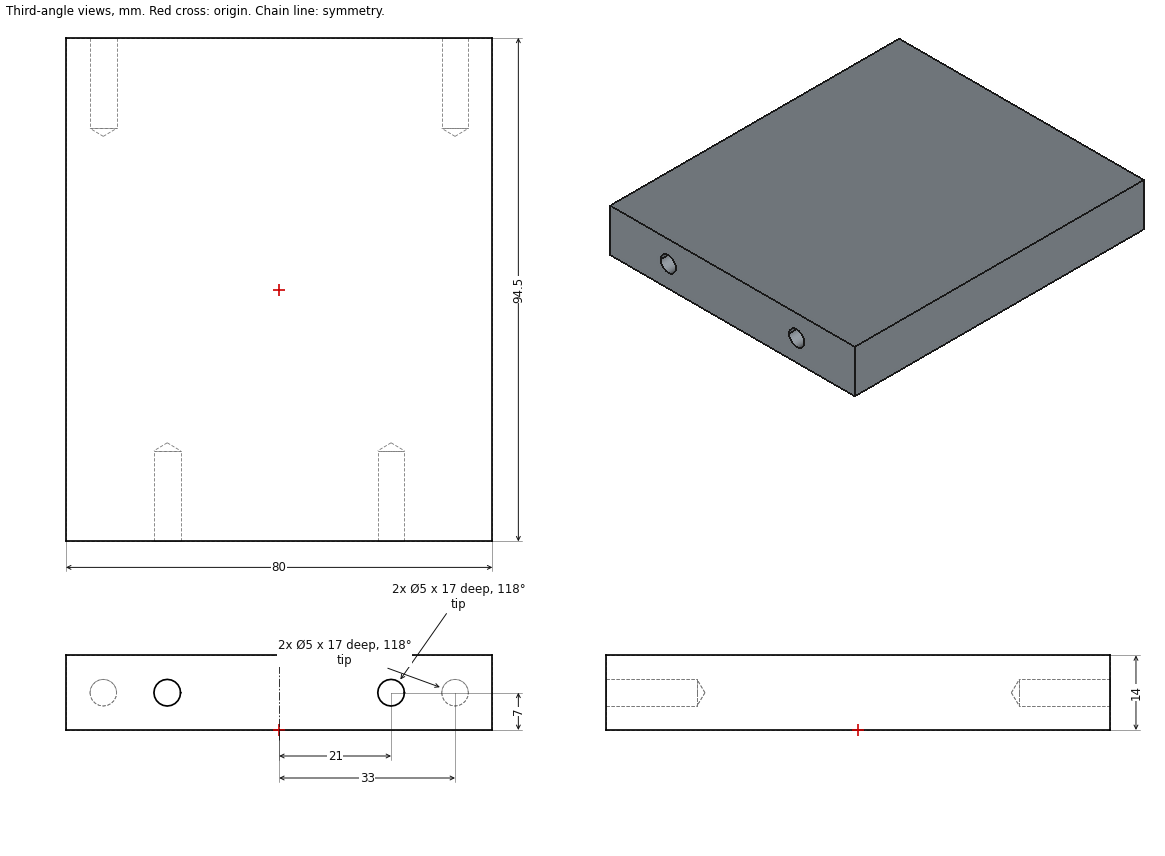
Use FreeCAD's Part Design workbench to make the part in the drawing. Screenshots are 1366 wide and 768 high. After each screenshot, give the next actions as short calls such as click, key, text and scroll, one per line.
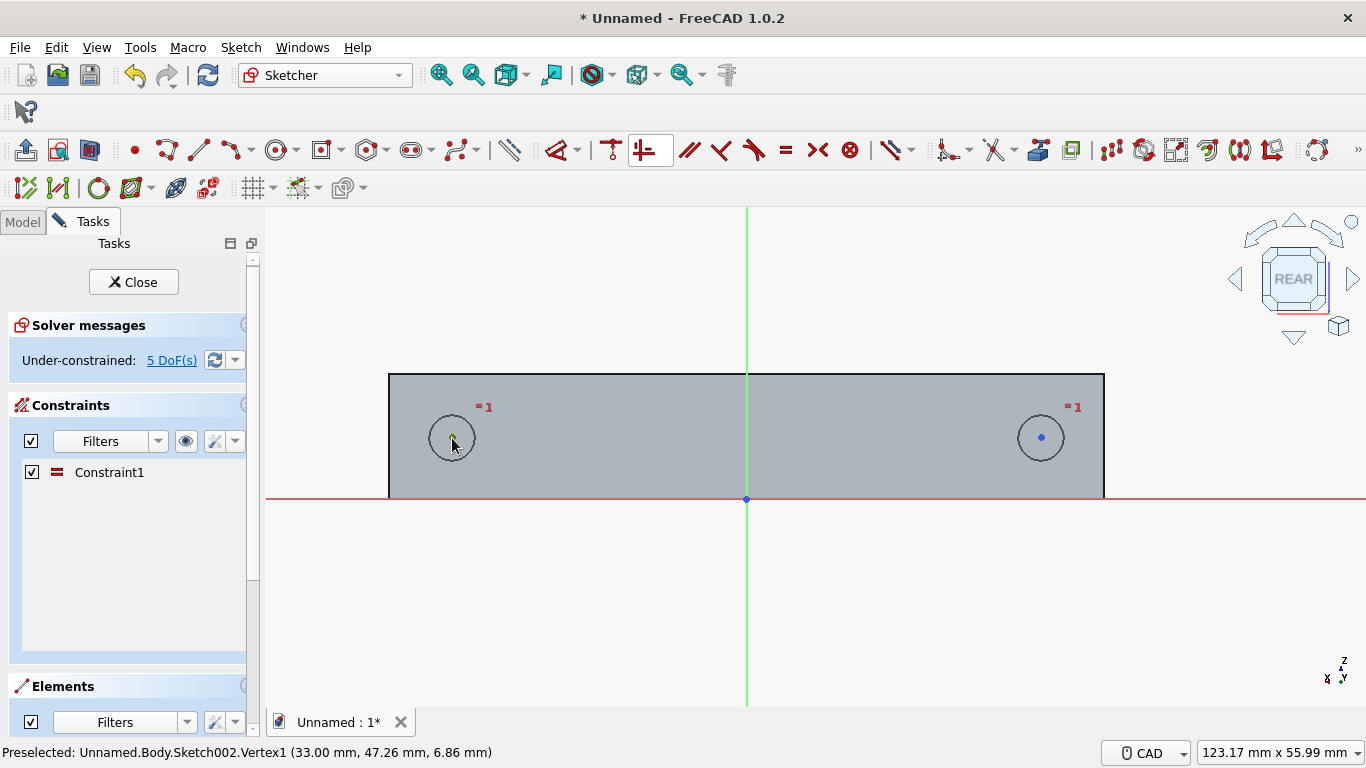
click(1041, 438)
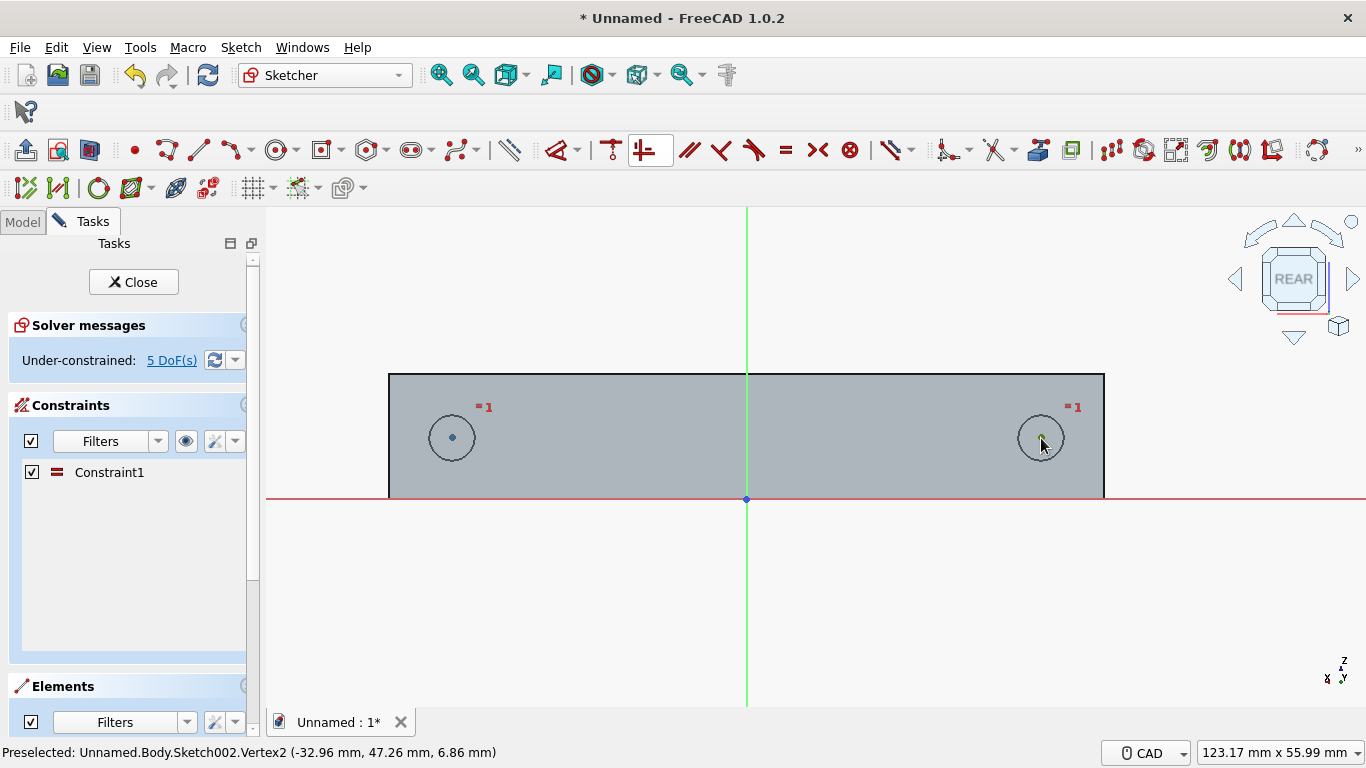
click(747, 647)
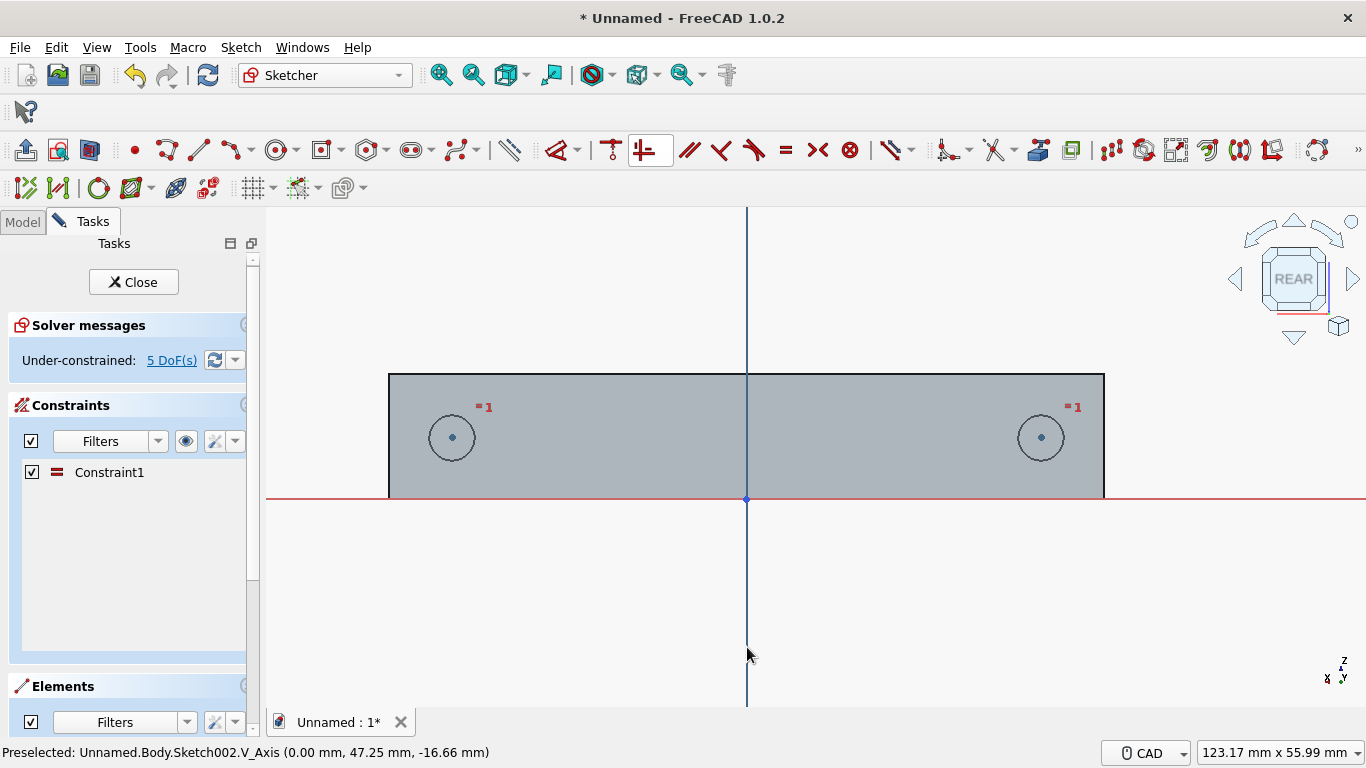
key(s)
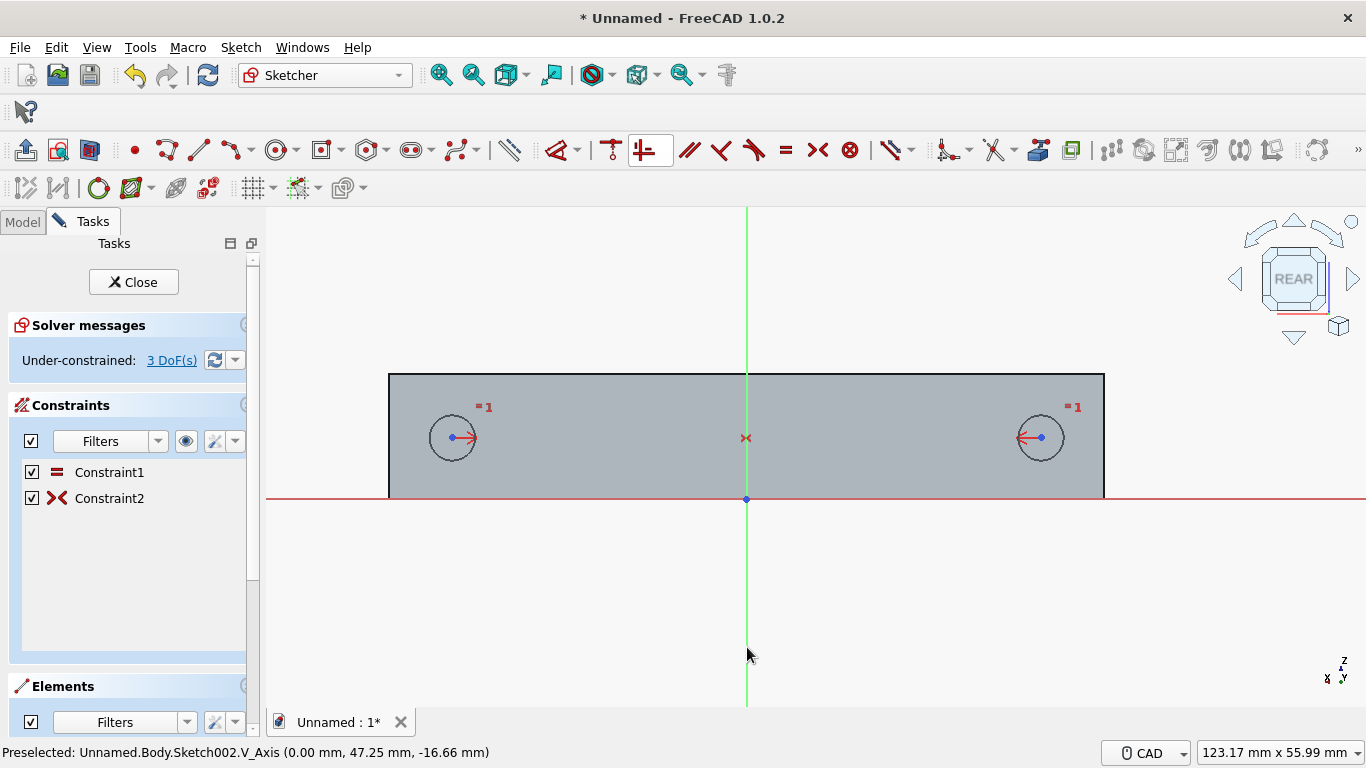
click(556, 150)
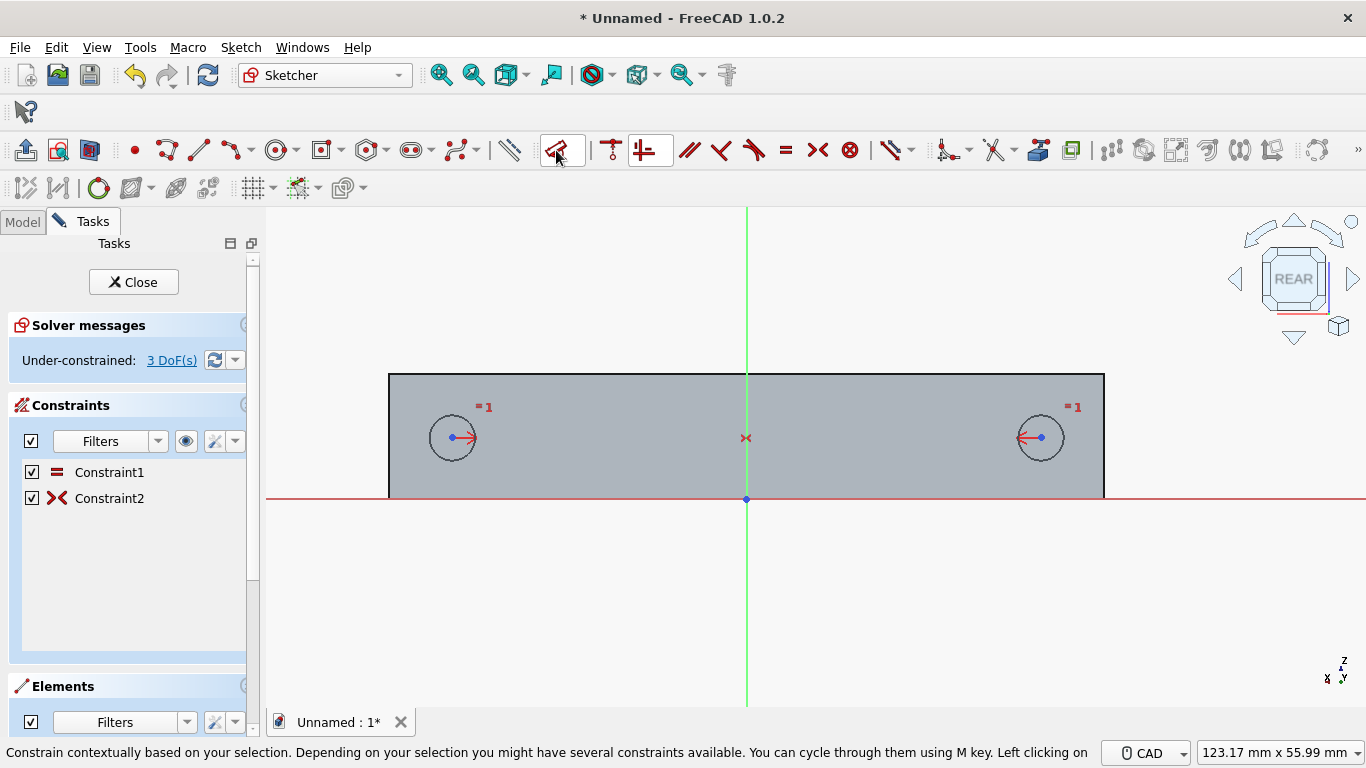
click(468, 422)
click(490, 399)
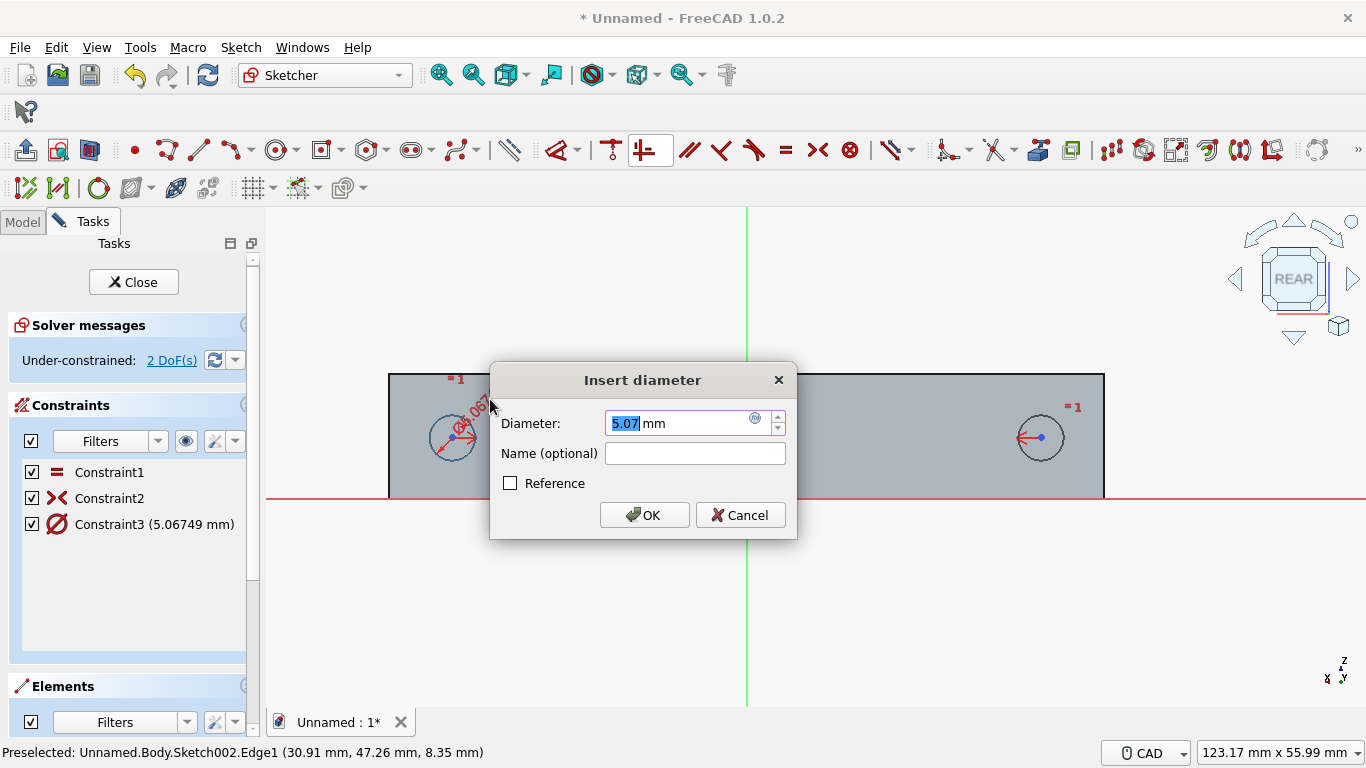
text(5)
key(Return)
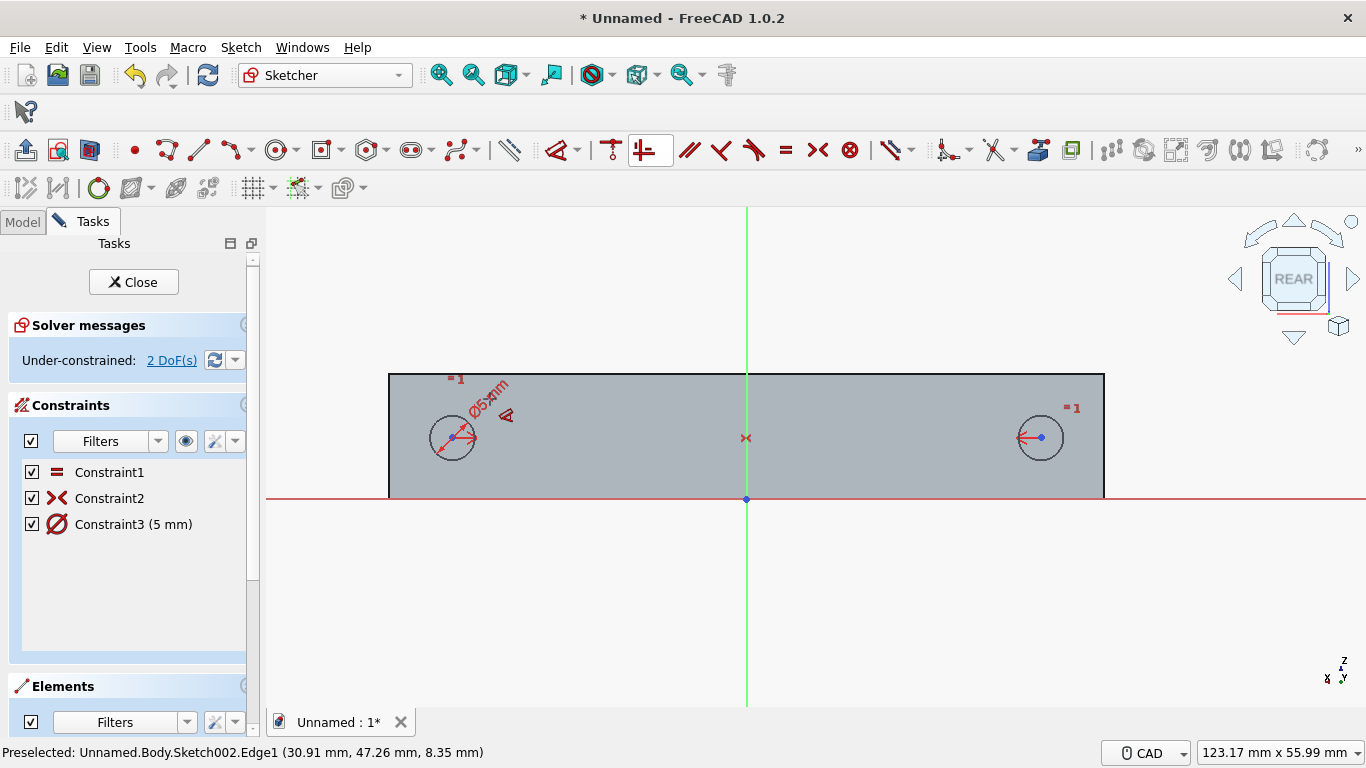
click(452, 438)
click(418, 469)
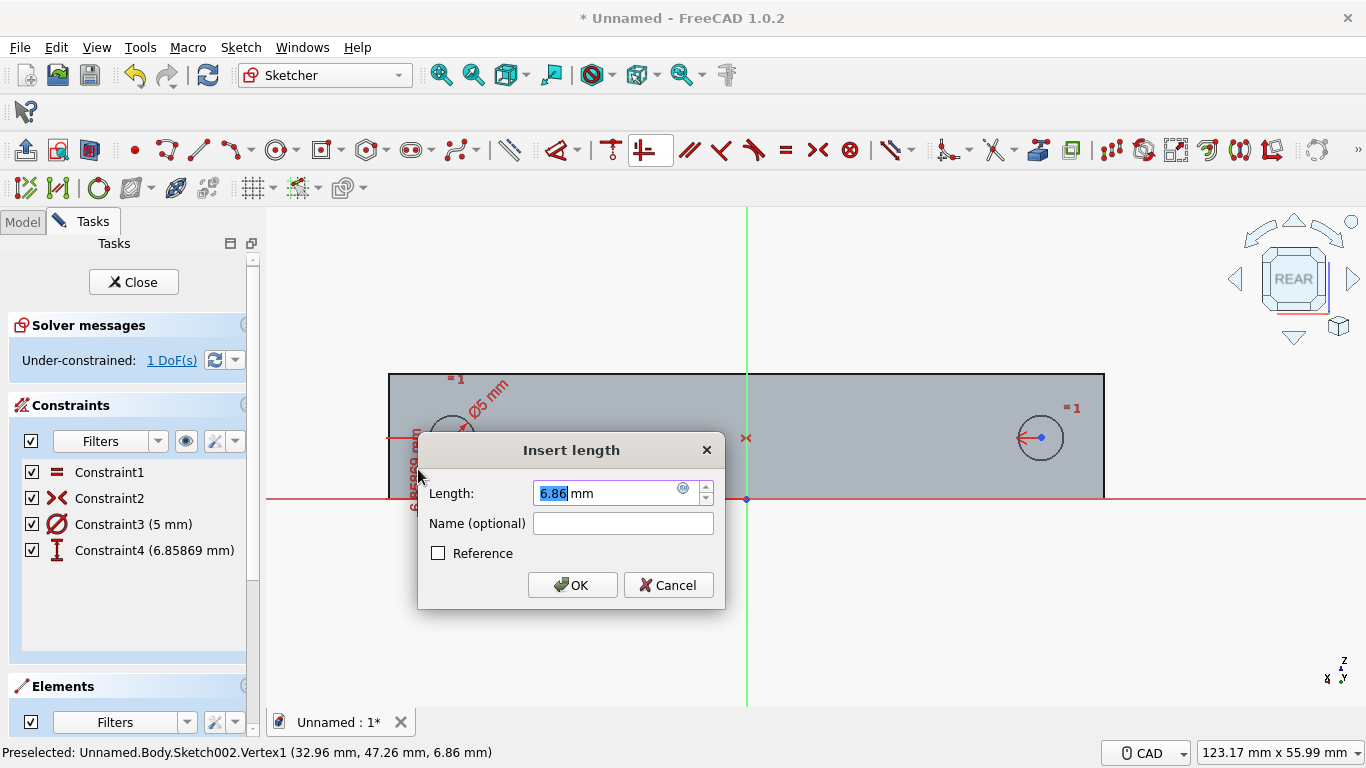
text(7)
key(Return)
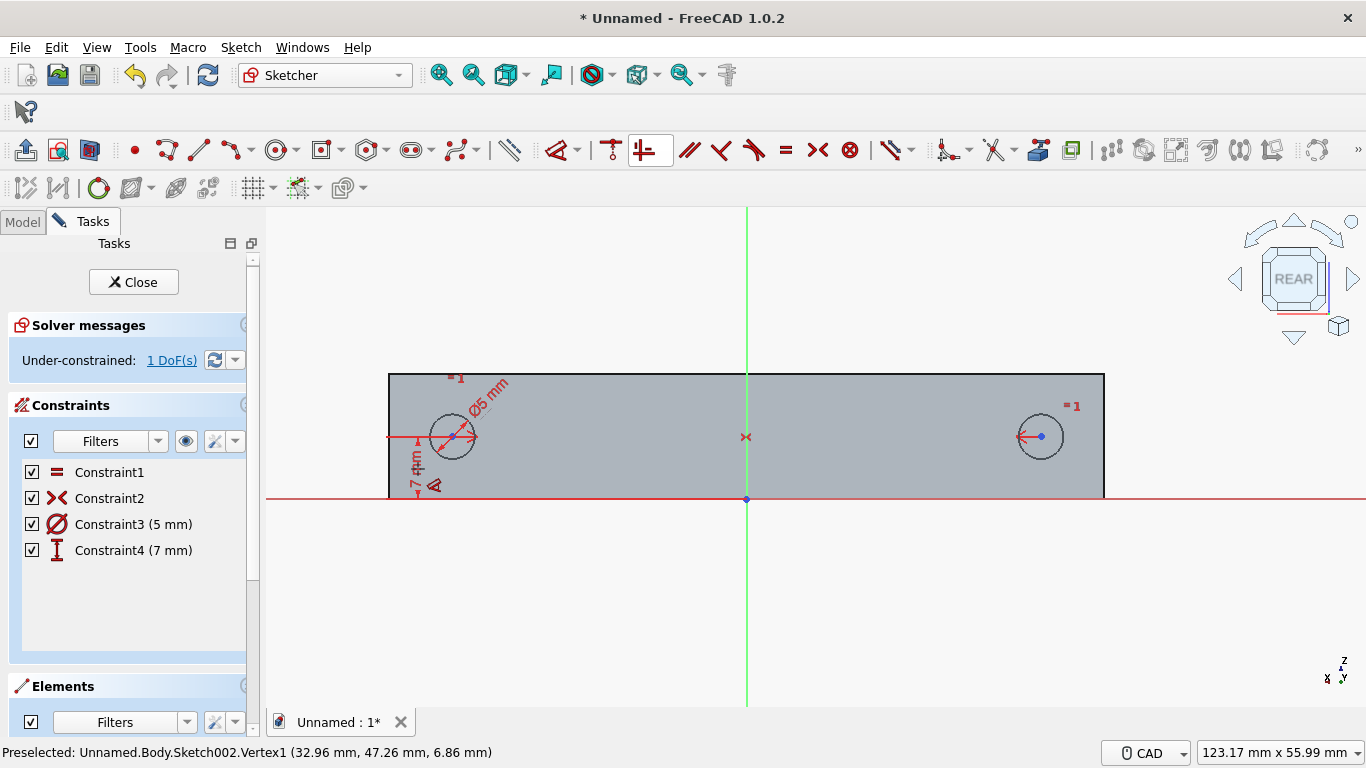
click(452, 437)
click(600, 533)